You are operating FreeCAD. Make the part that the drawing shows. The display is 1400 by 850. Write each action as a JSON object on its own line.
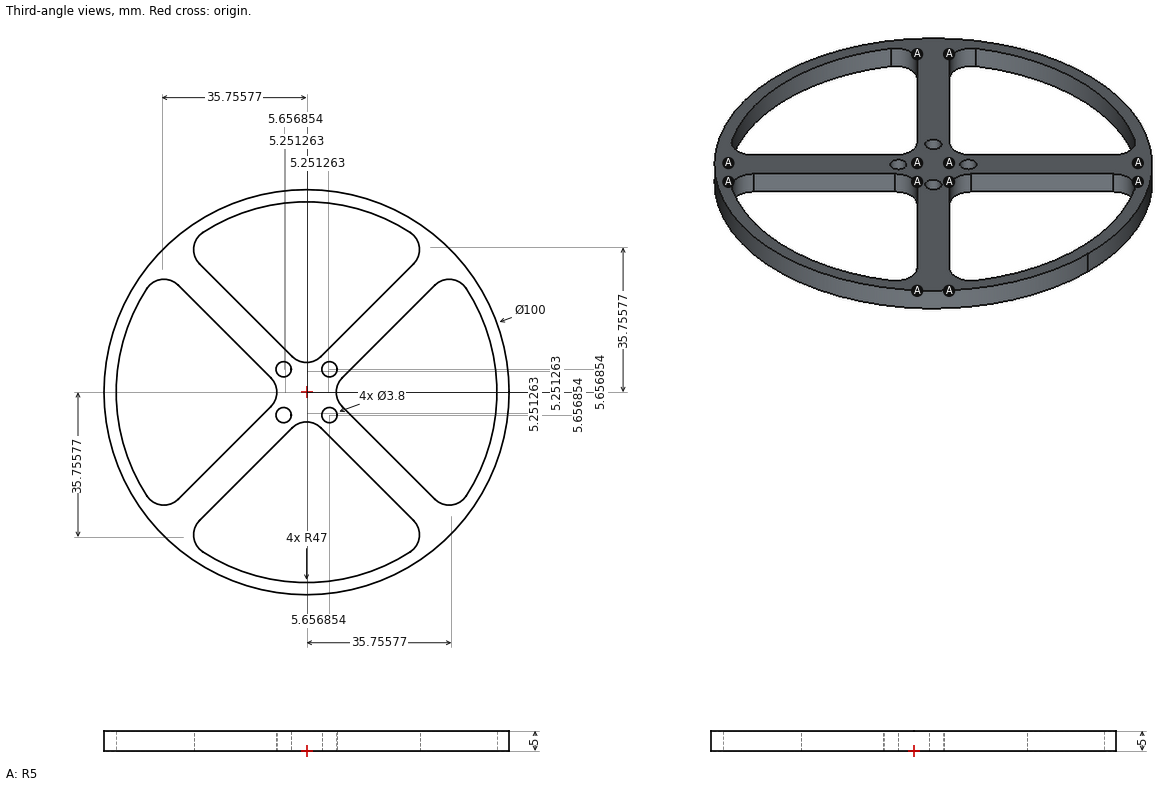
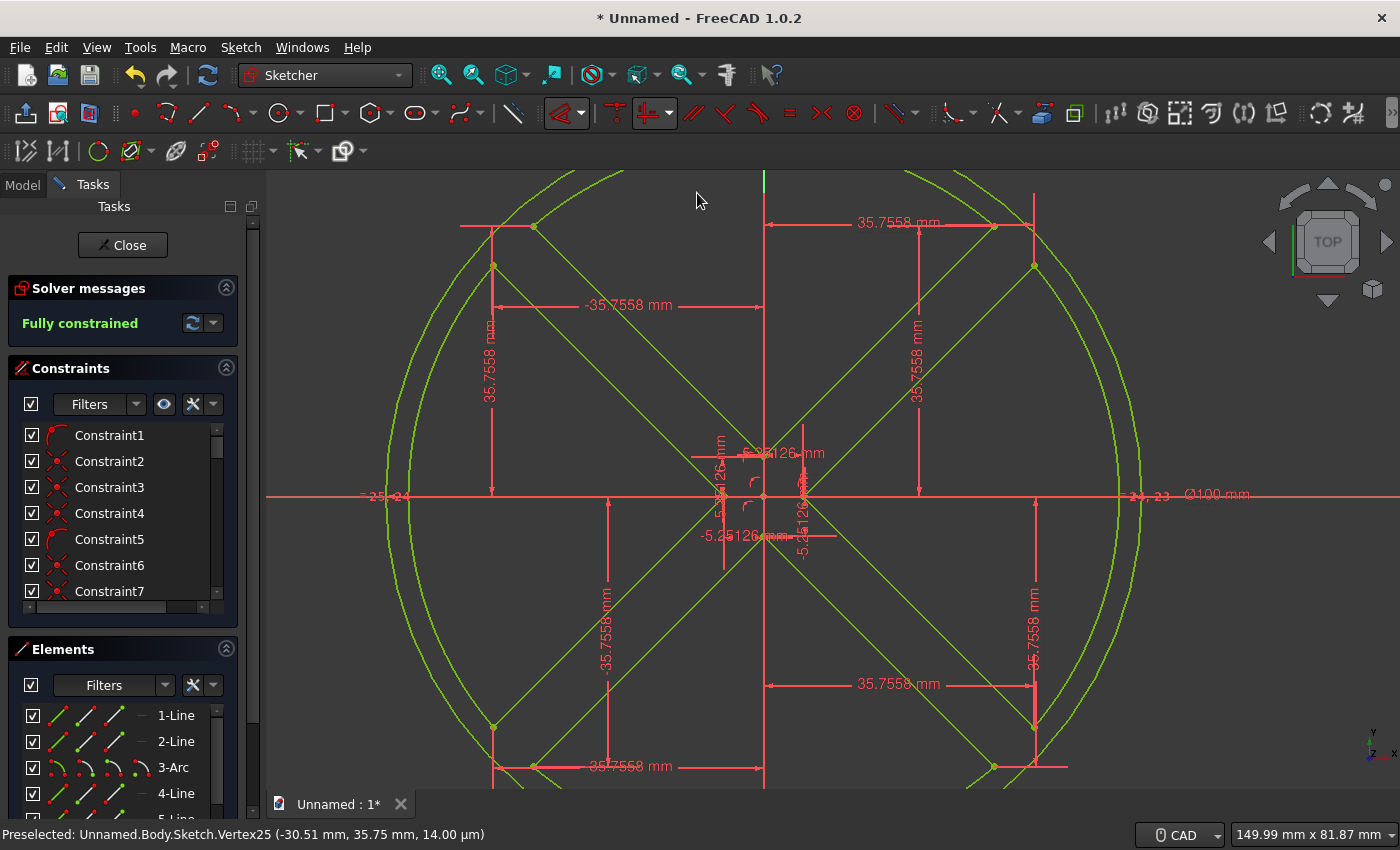
{"action": "left_click", "coordinate": [123, 245]}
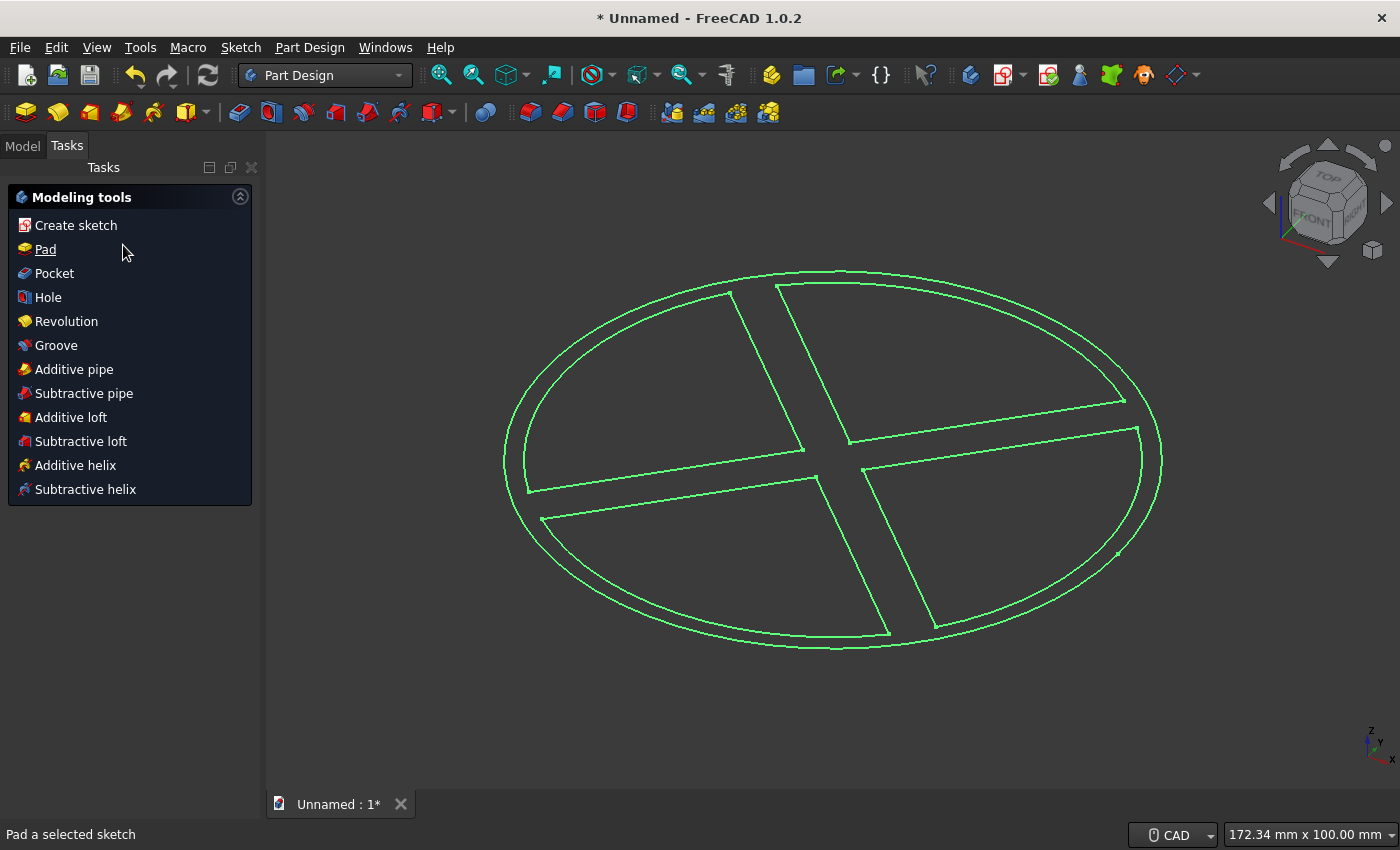
{"action": "left_click", "coordinate": [26, 112]}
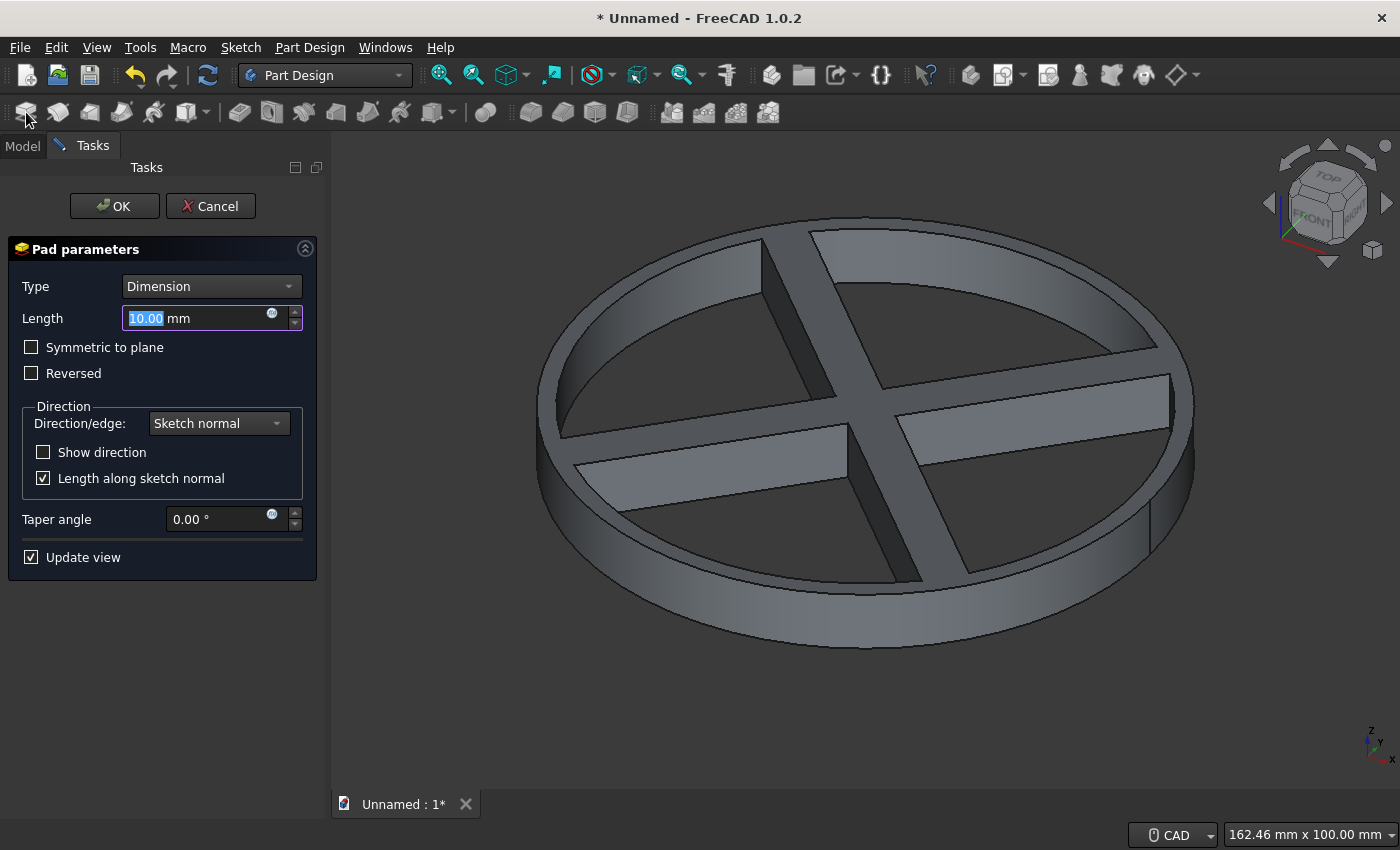
{"action": "type", "text": "5"}
{"action": "key", "text": "Tab"}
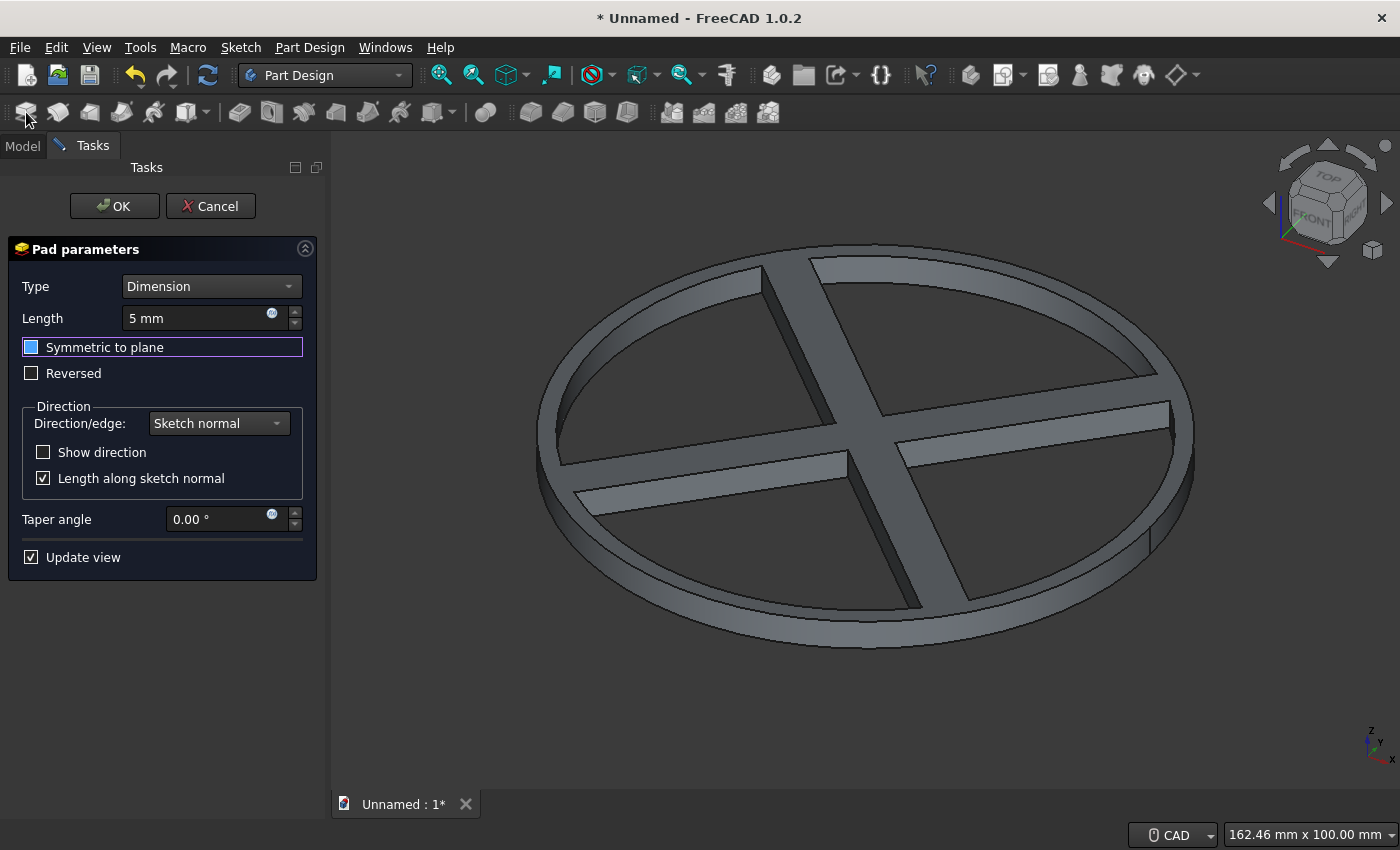
{"action": "left_click", "coordinate": [115, 206]}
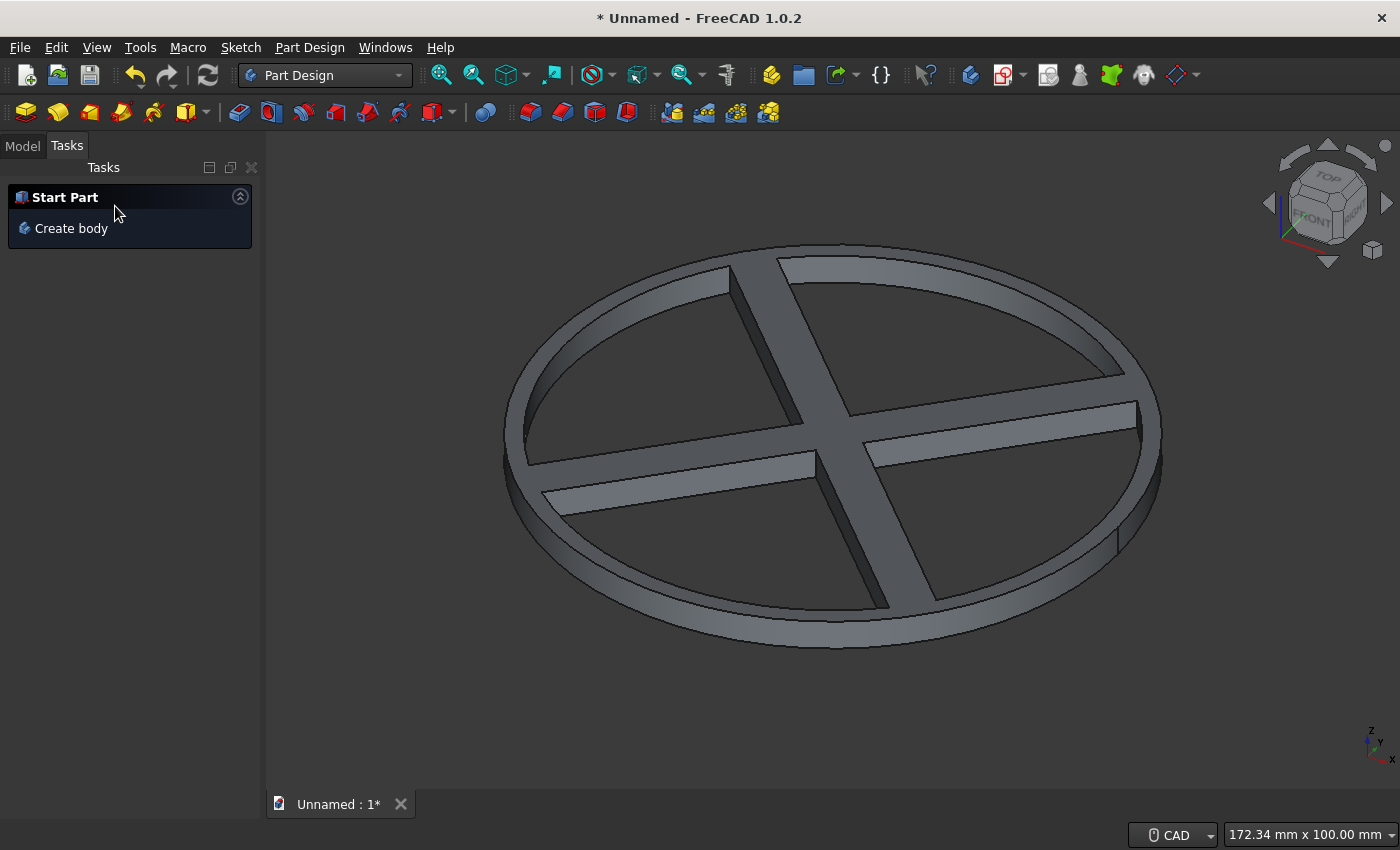
{"action": "key", "text": "0"}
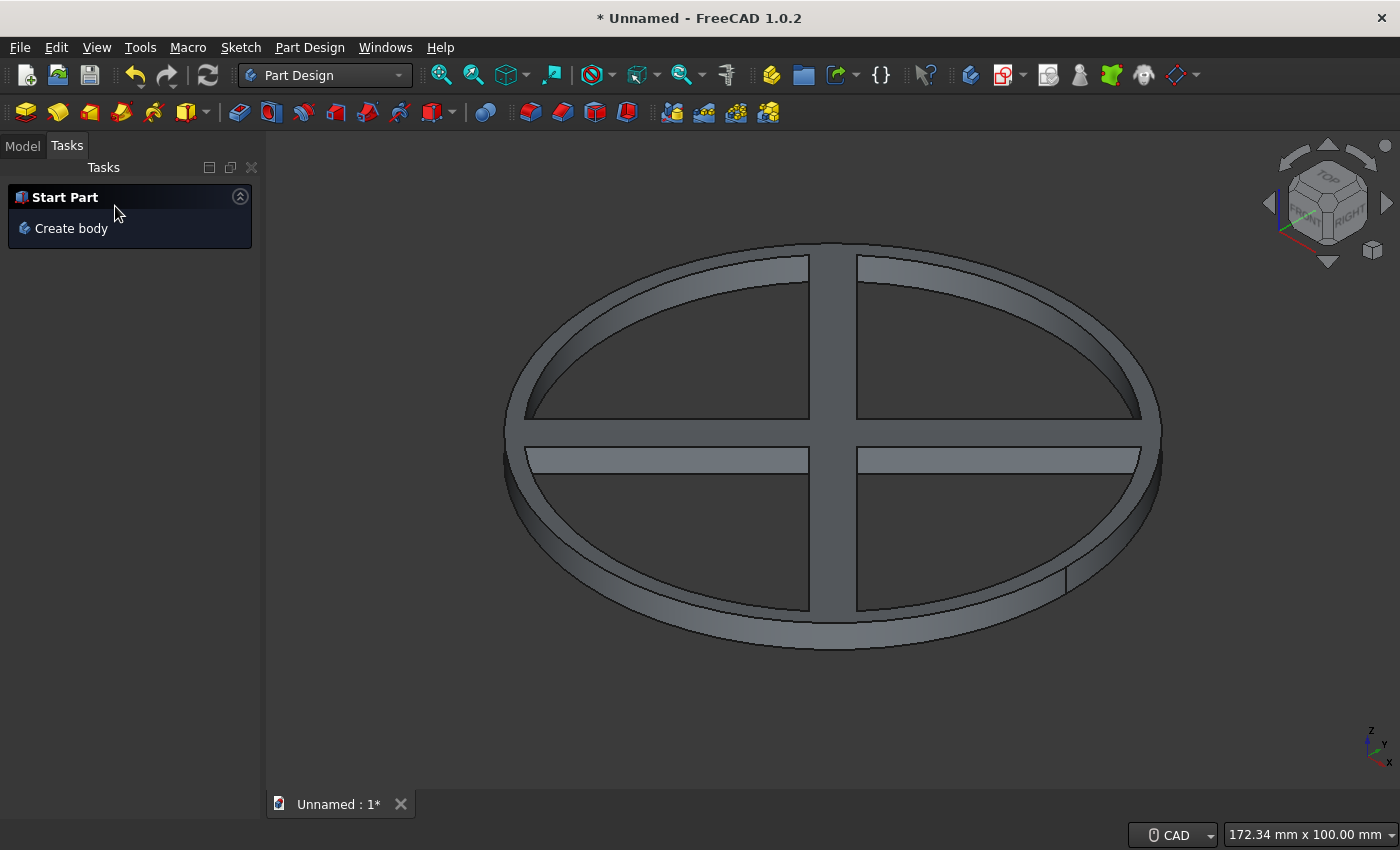
{"action": "key", "text": "2"}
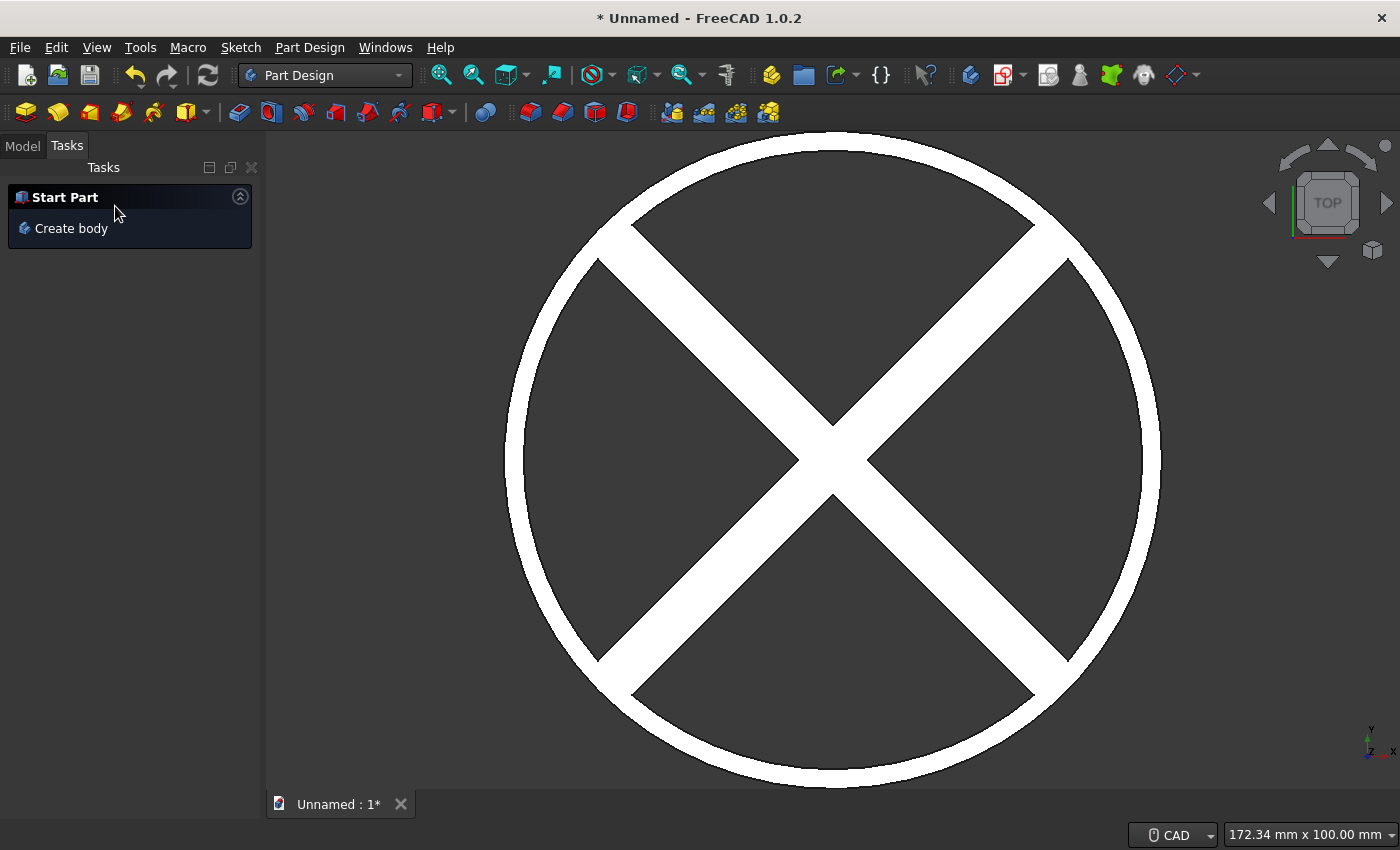
{"action": "left_click", "coordinate": [442, 76]}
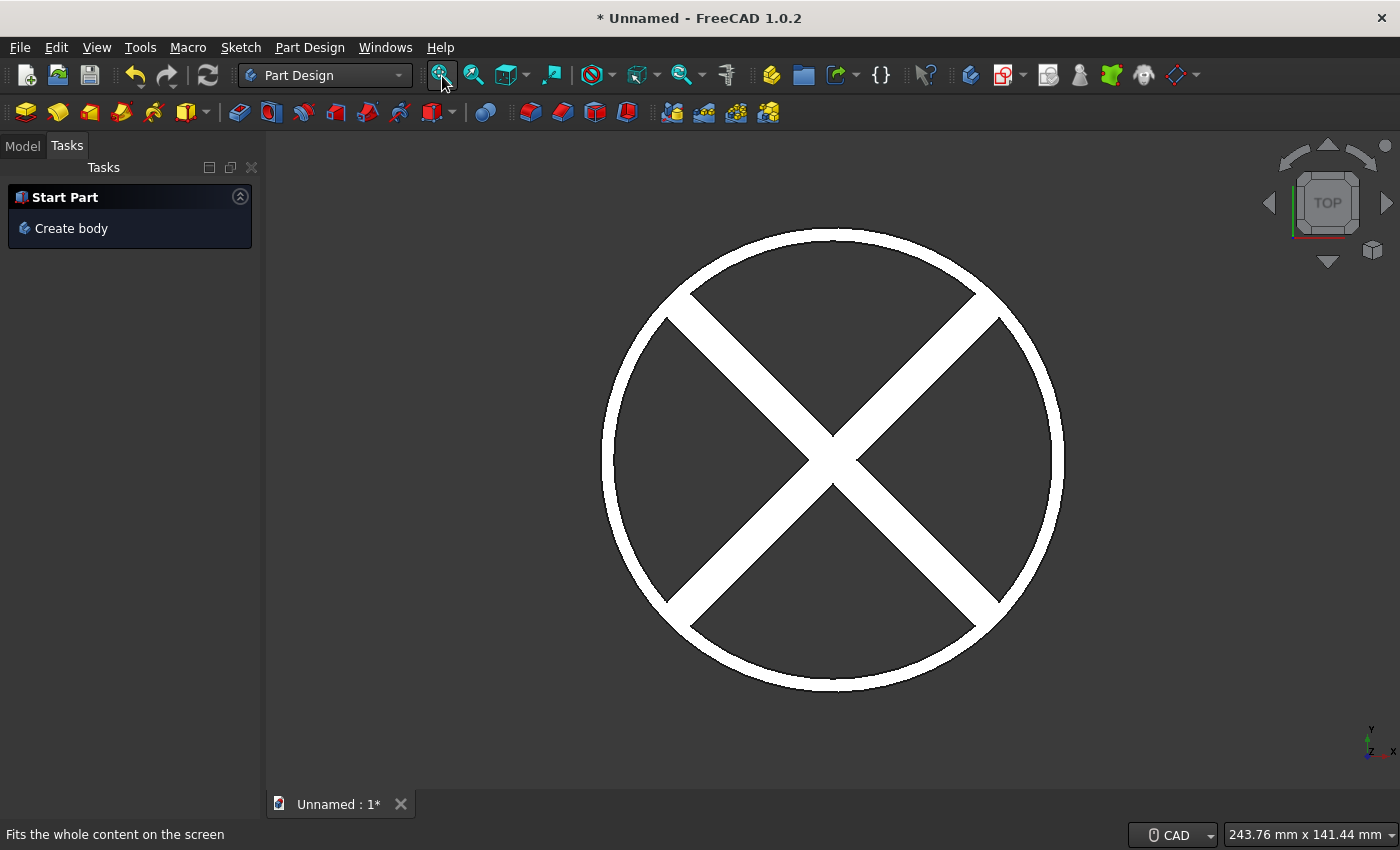
{"action": "key", "text": "1"}